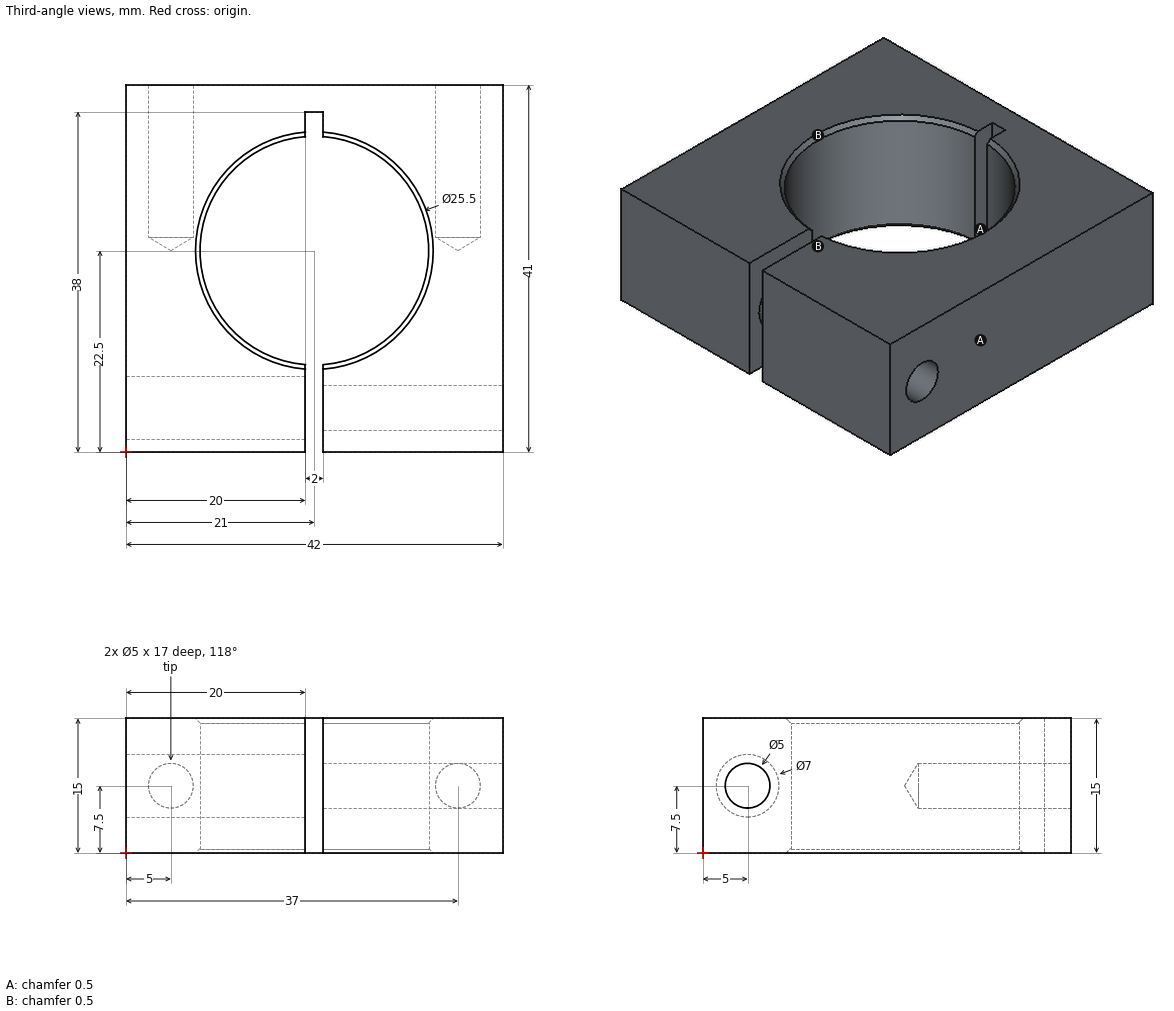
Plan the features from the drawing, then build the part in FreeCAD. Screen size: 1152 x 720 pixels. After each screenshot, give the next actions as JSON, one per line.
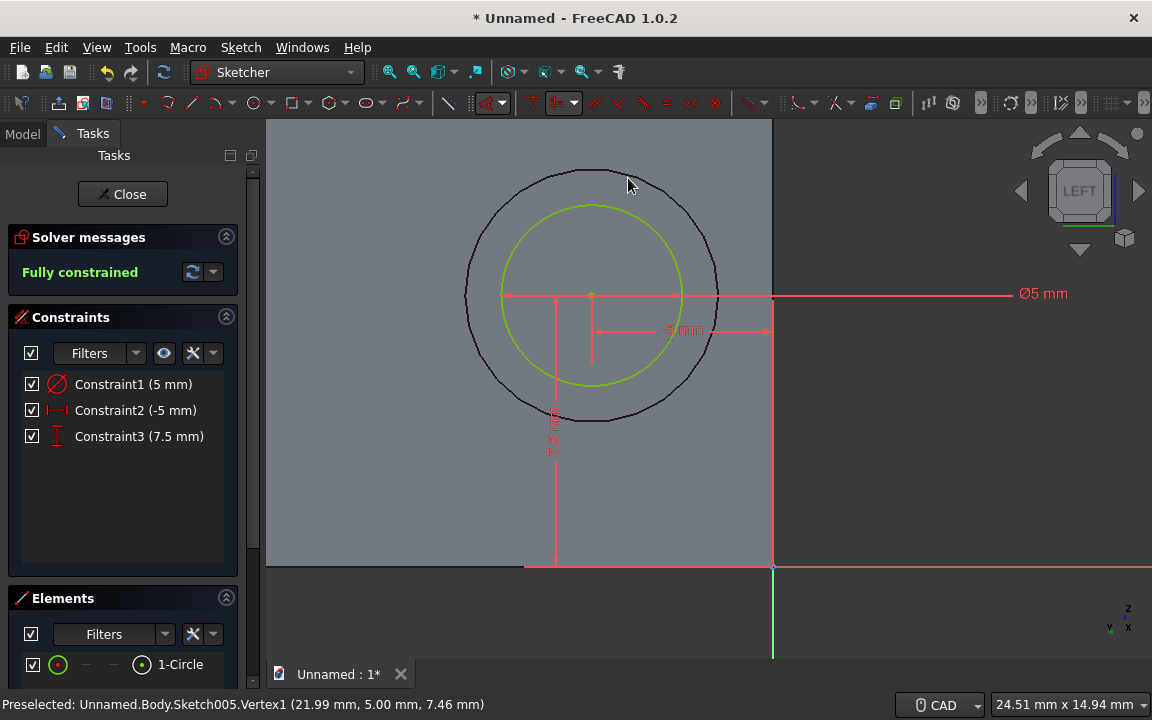
{"action": "left_click", "coordinate": [123, 194]}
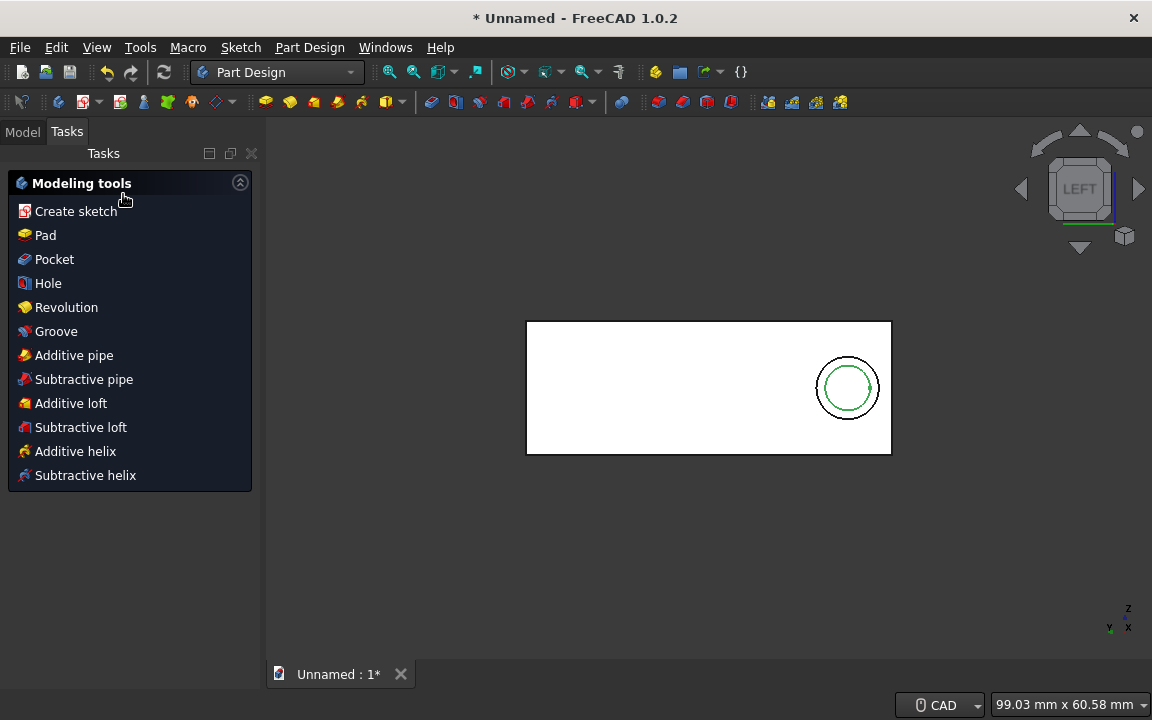
{"action": "left_click", "coordinate": [432, 102]}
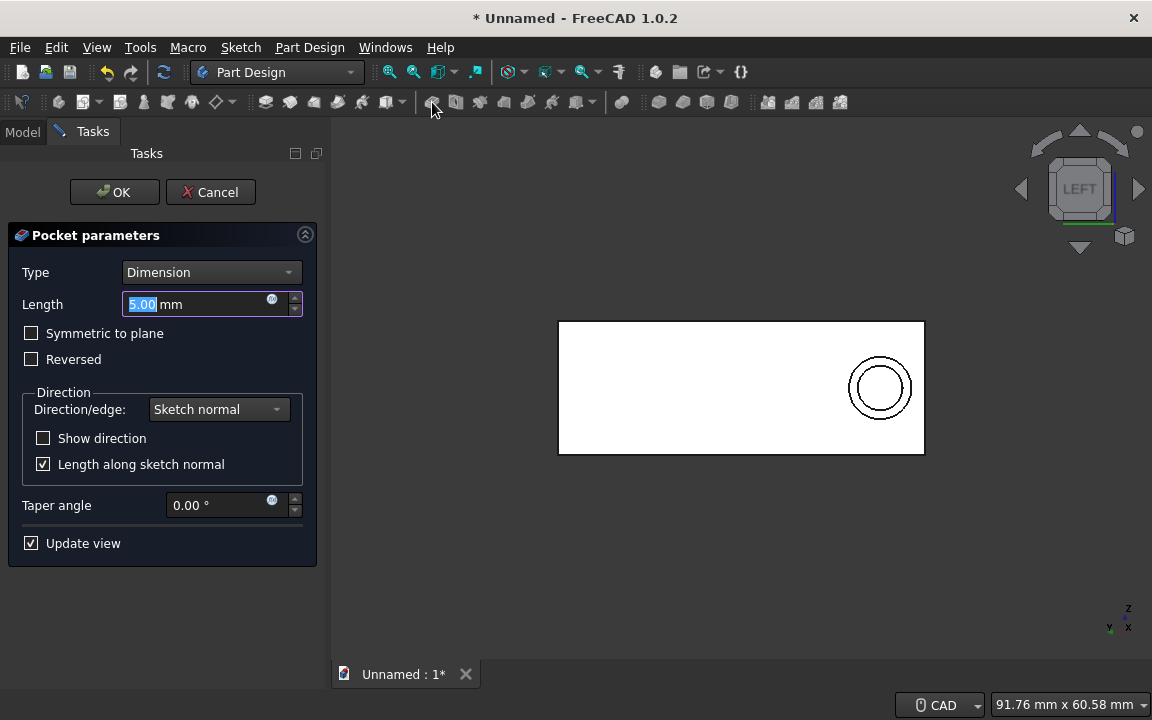
{"action": "left_click", "coordinate": [212, 272]}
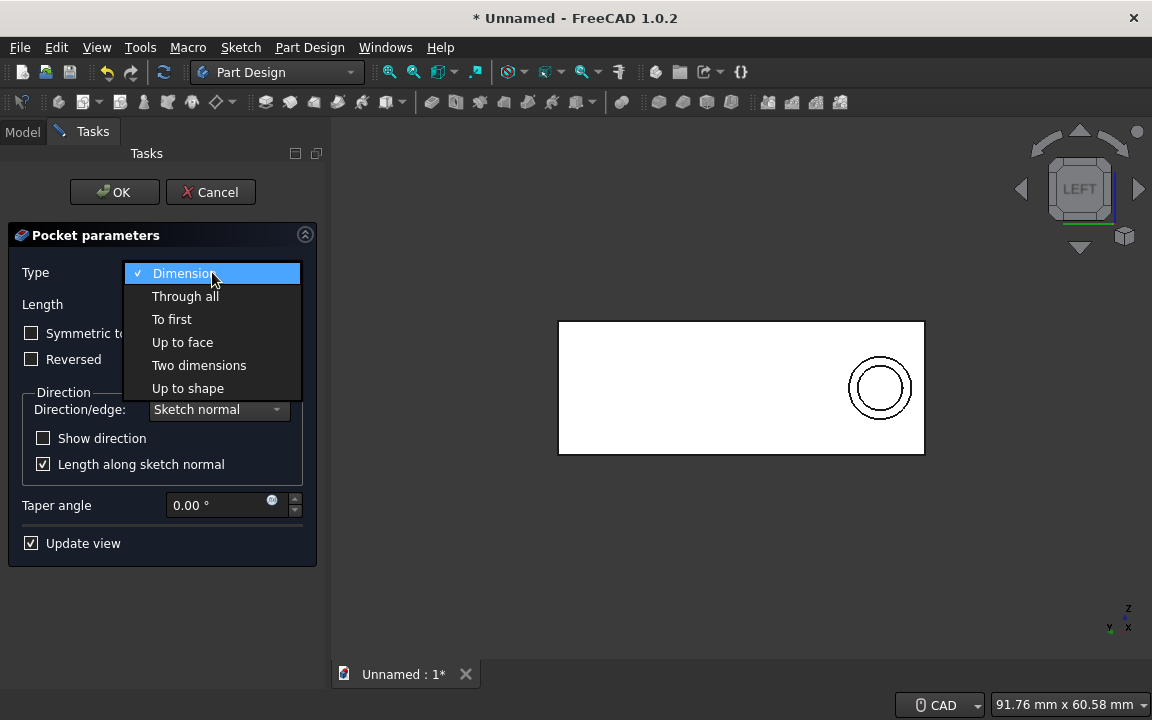
{"action": "left_click", "coordinate": [212, 296]}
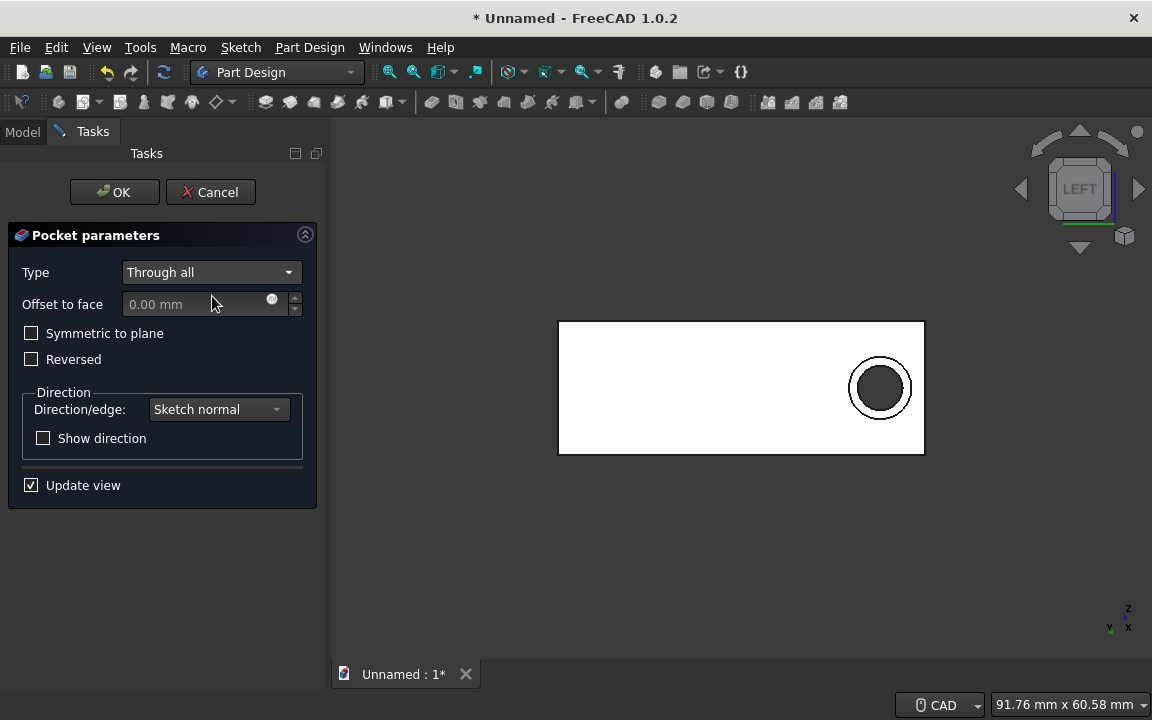
{"action": "left_click", "coordinate": [115, 192]}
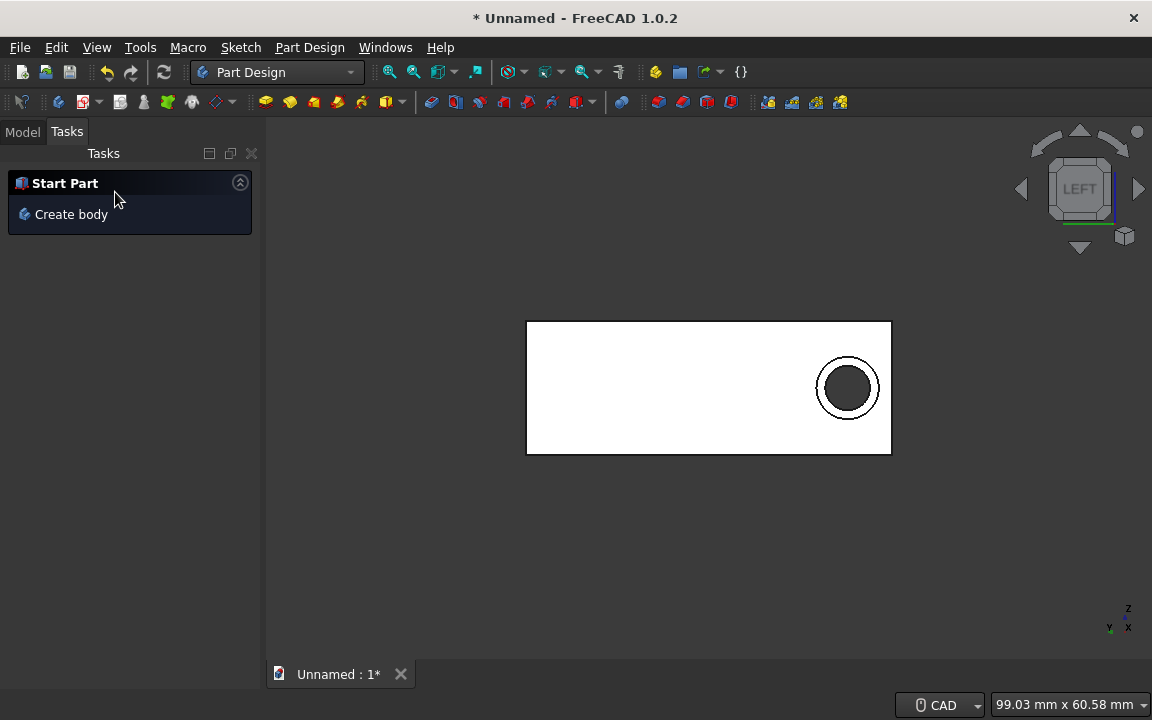
{"action": "left_click", "coordinate": [390, 72]}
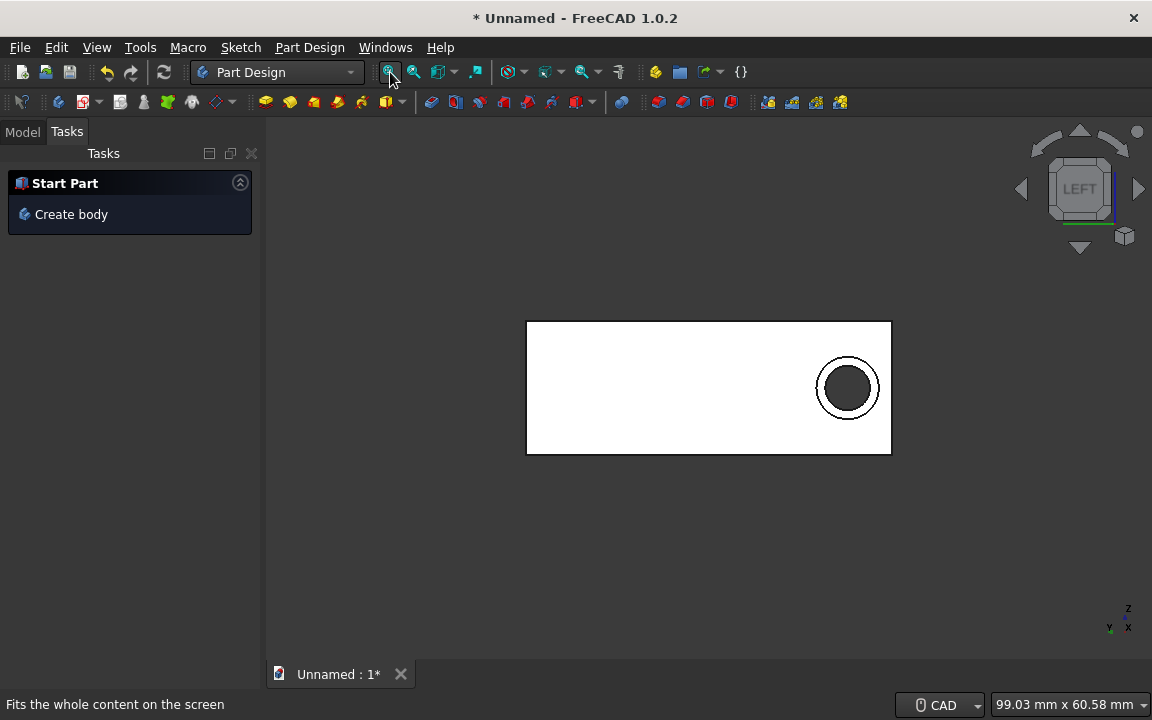
{"action": "key", "text": "0"}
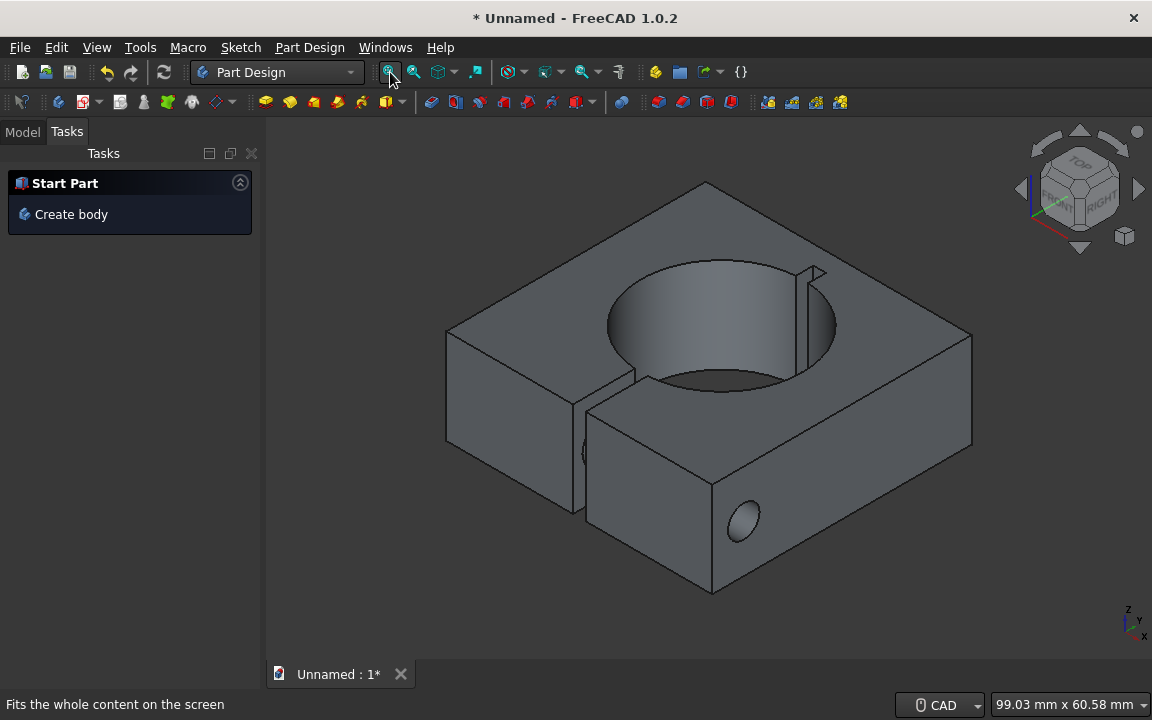
{"action": "key", "text": "2"}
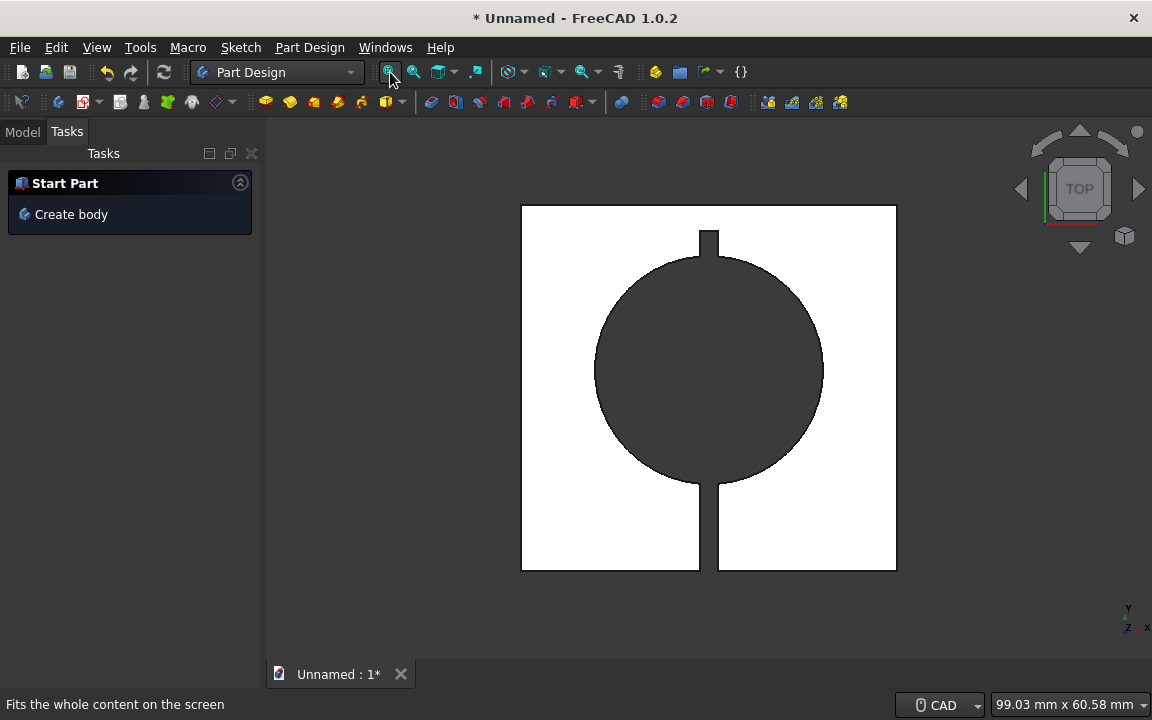
{"action": "left_click", "coordinate": [793, 447]}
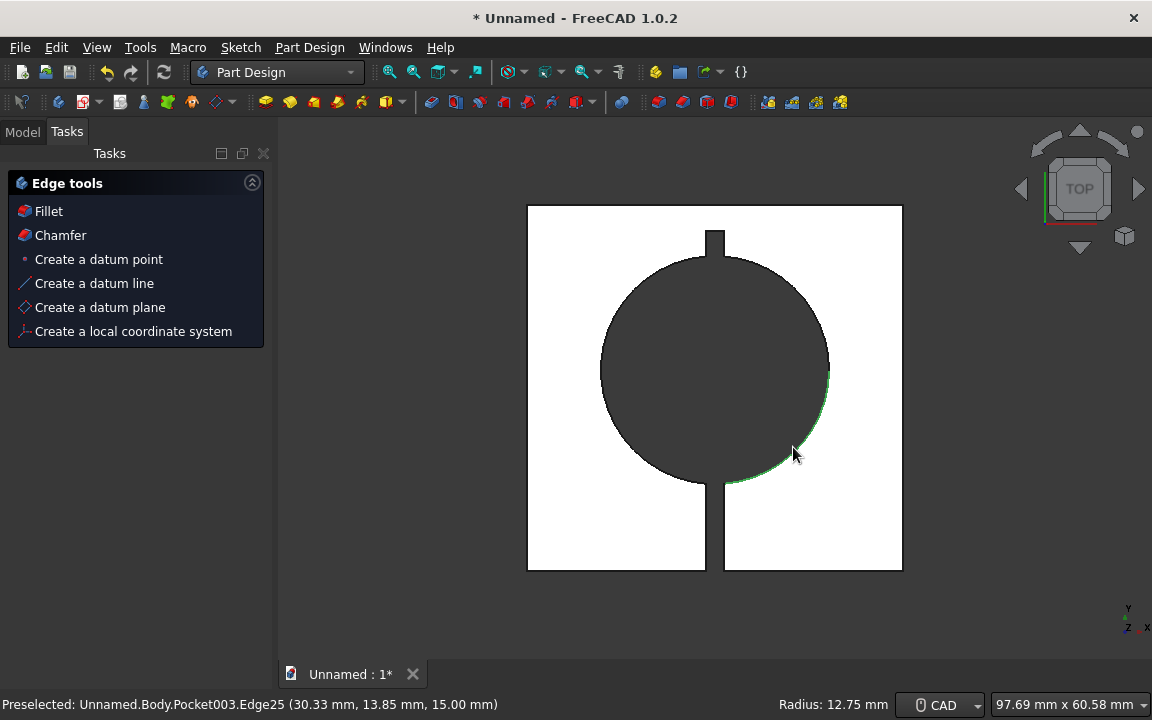
{"action": "key", "text": "1"}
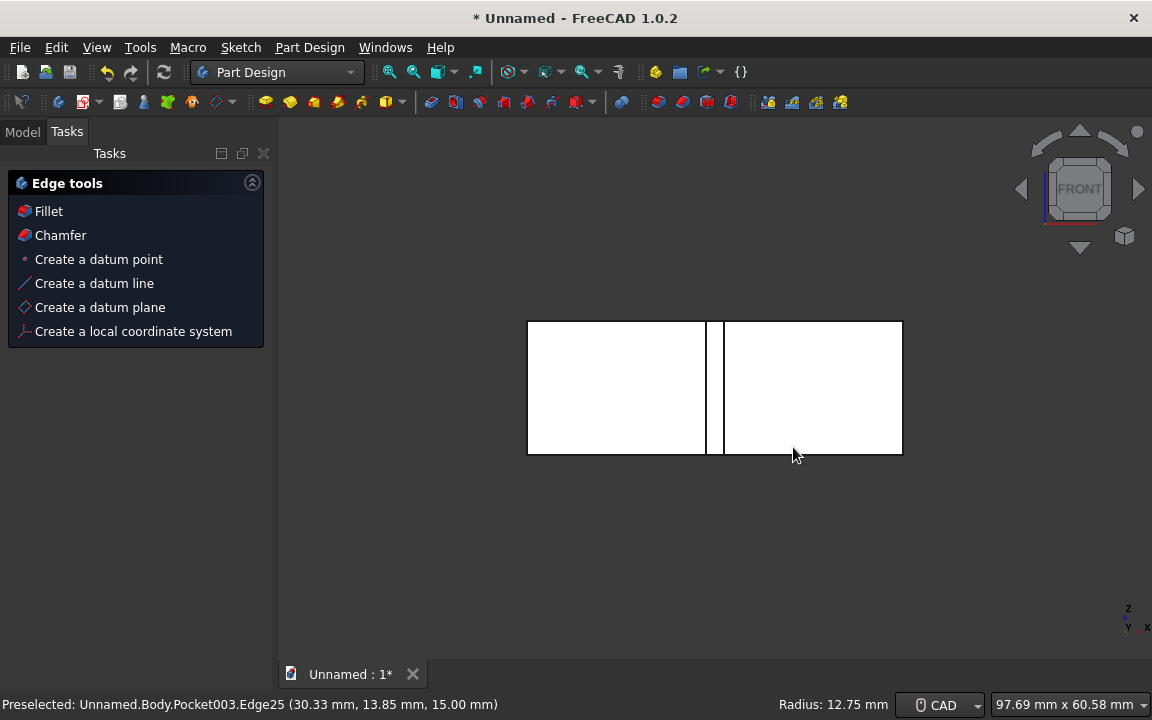
{"action": "left_click", "coordinate": [390, 72]}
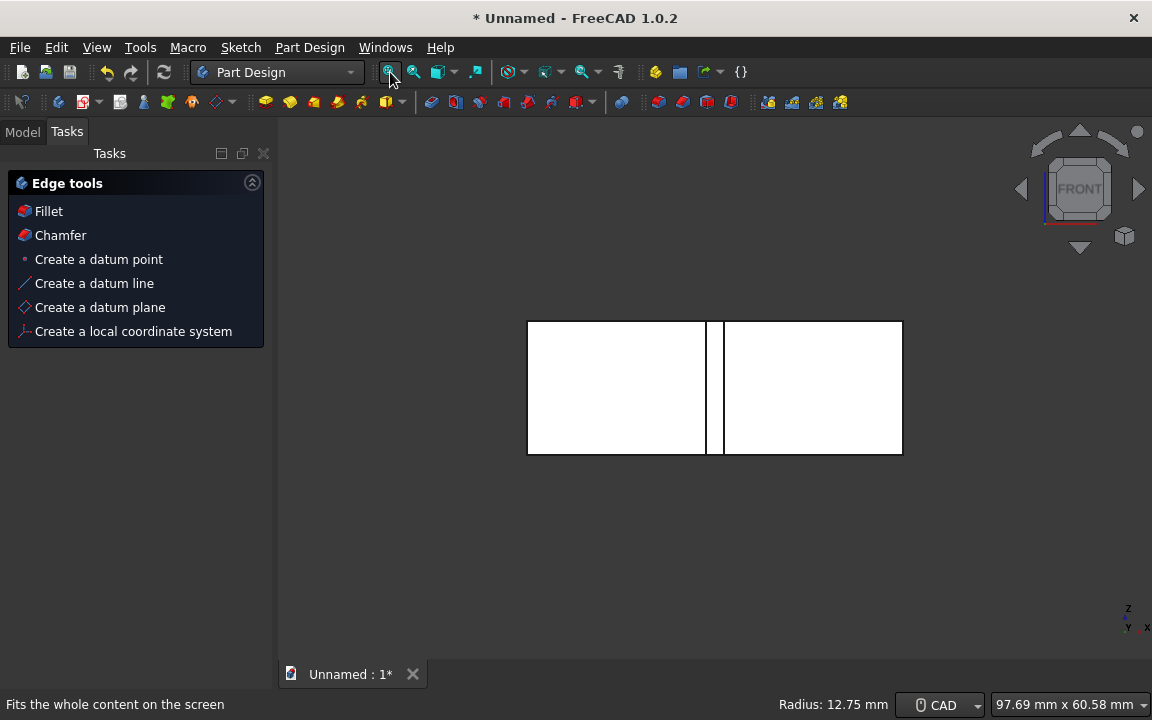
{"action": "key", "text": "3"}